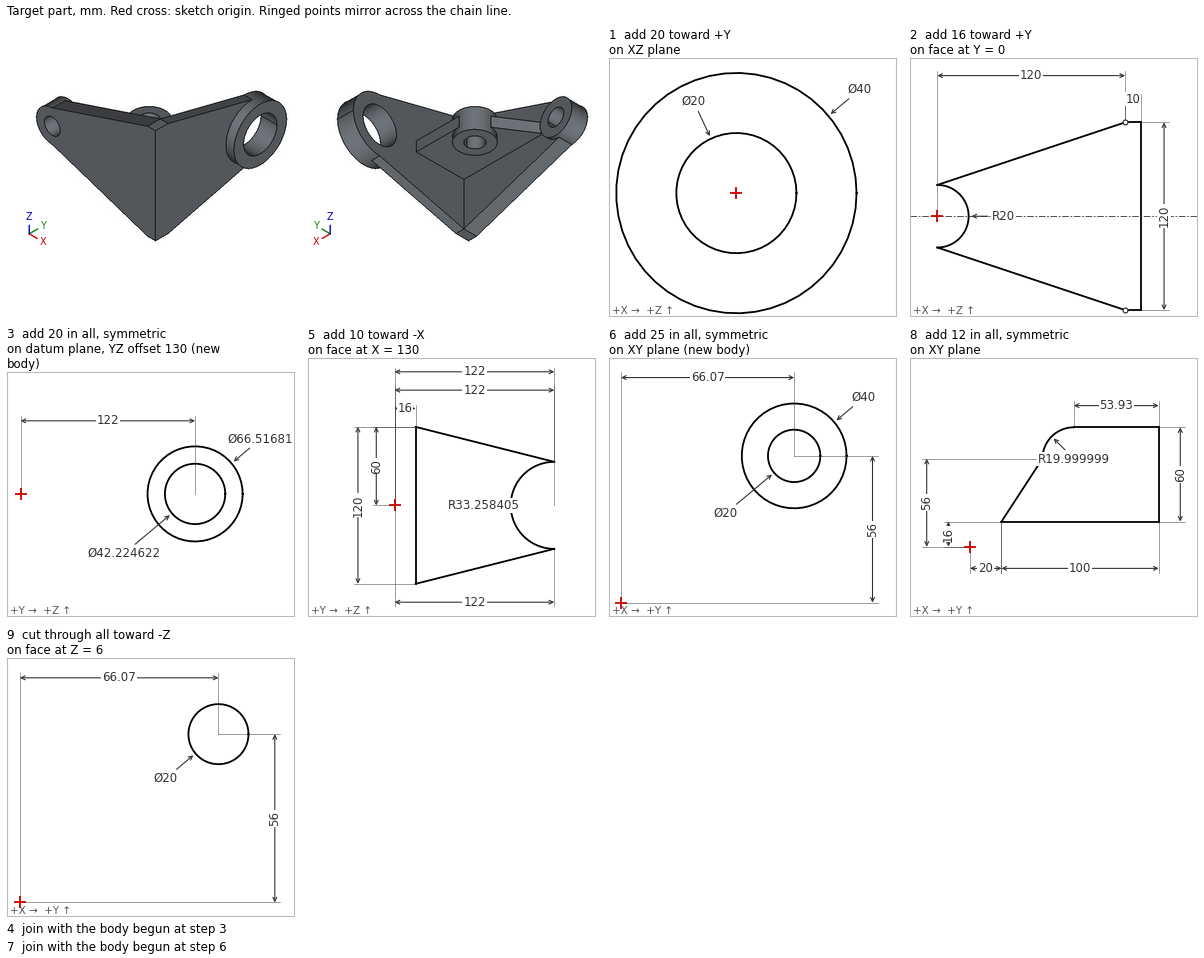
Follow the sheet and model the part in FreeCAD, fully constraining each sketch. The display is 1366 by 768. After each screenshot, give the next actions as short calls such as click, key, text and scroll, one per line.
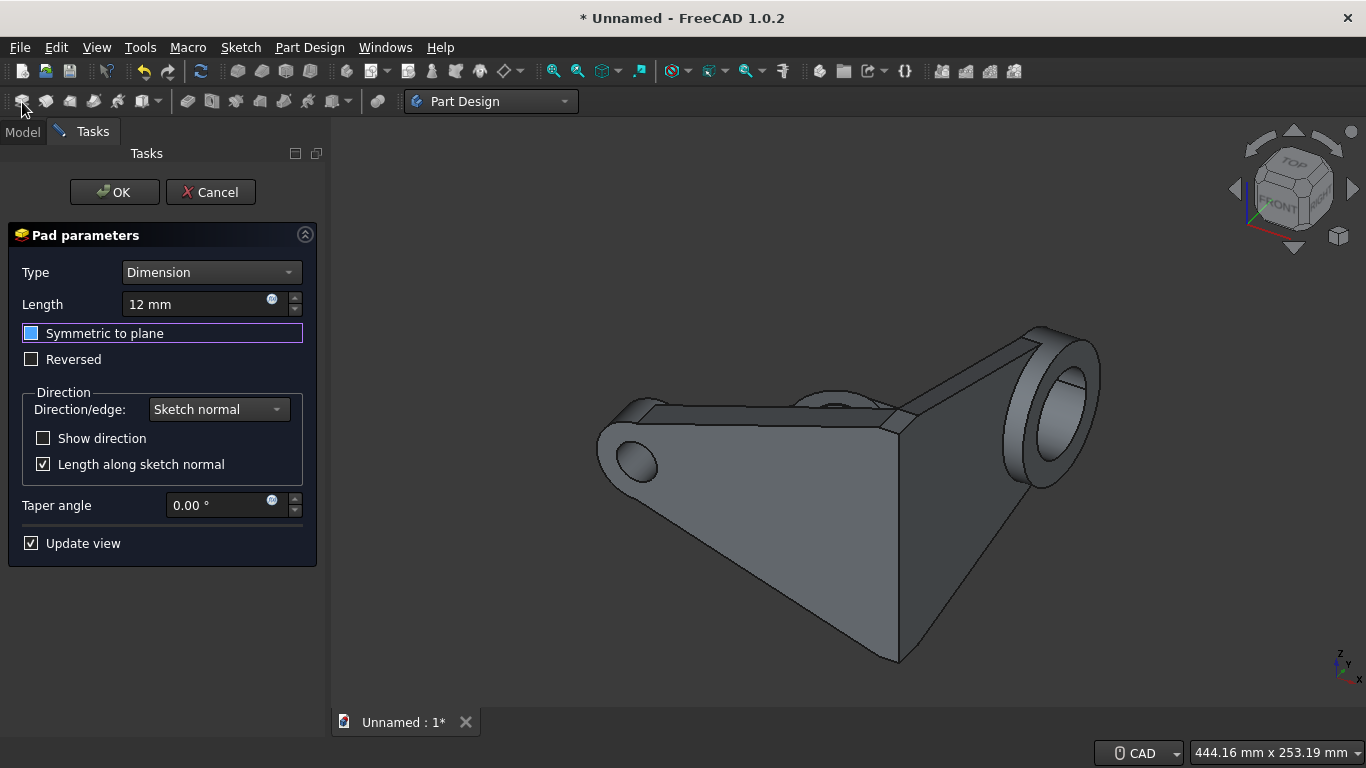
click(30, 333)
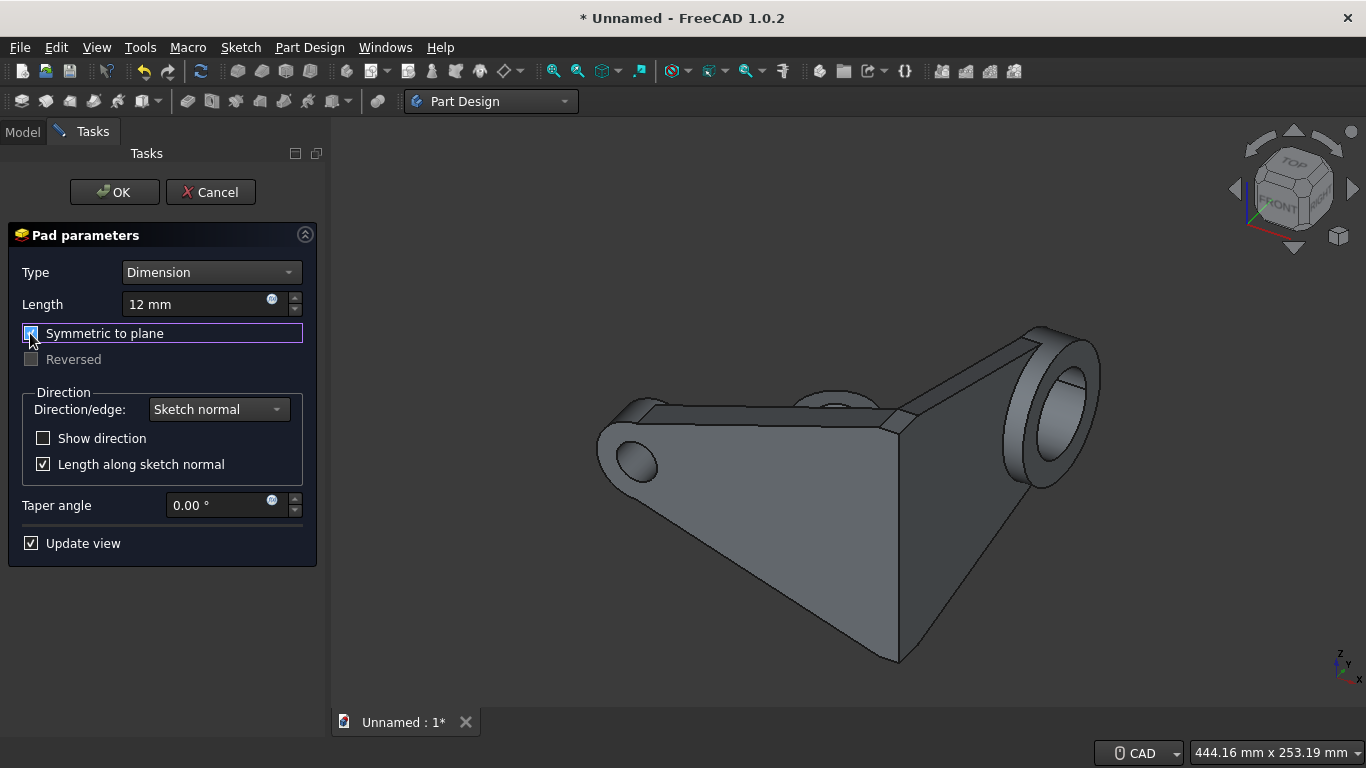
click(115, 192)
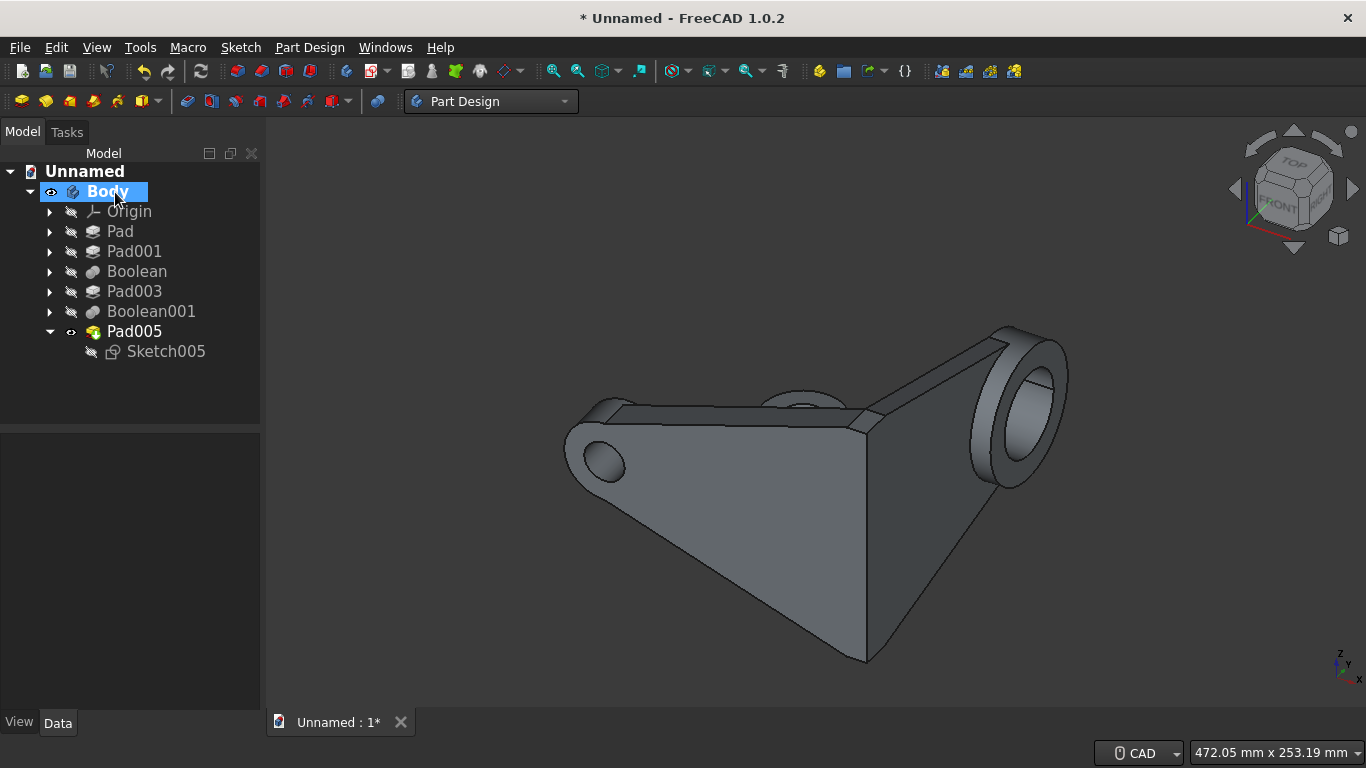
key(0)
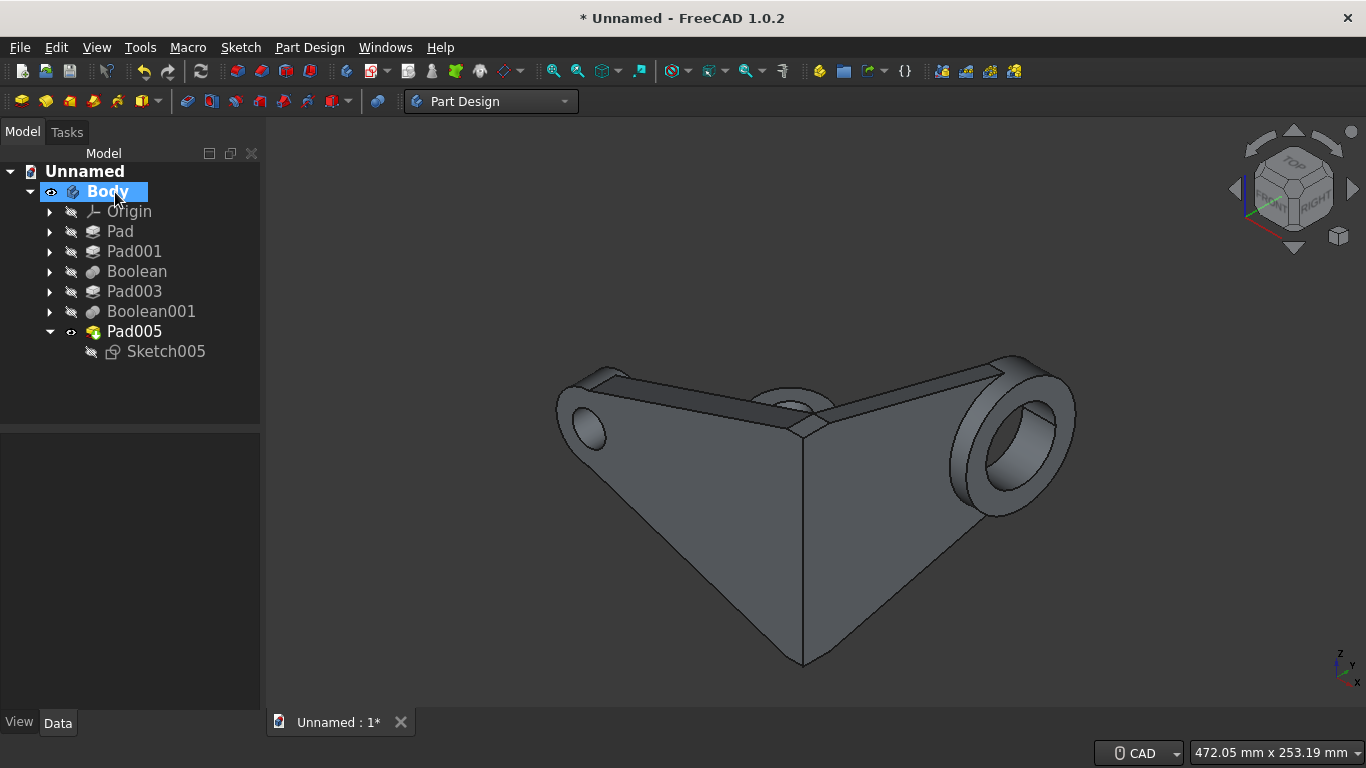
key(2)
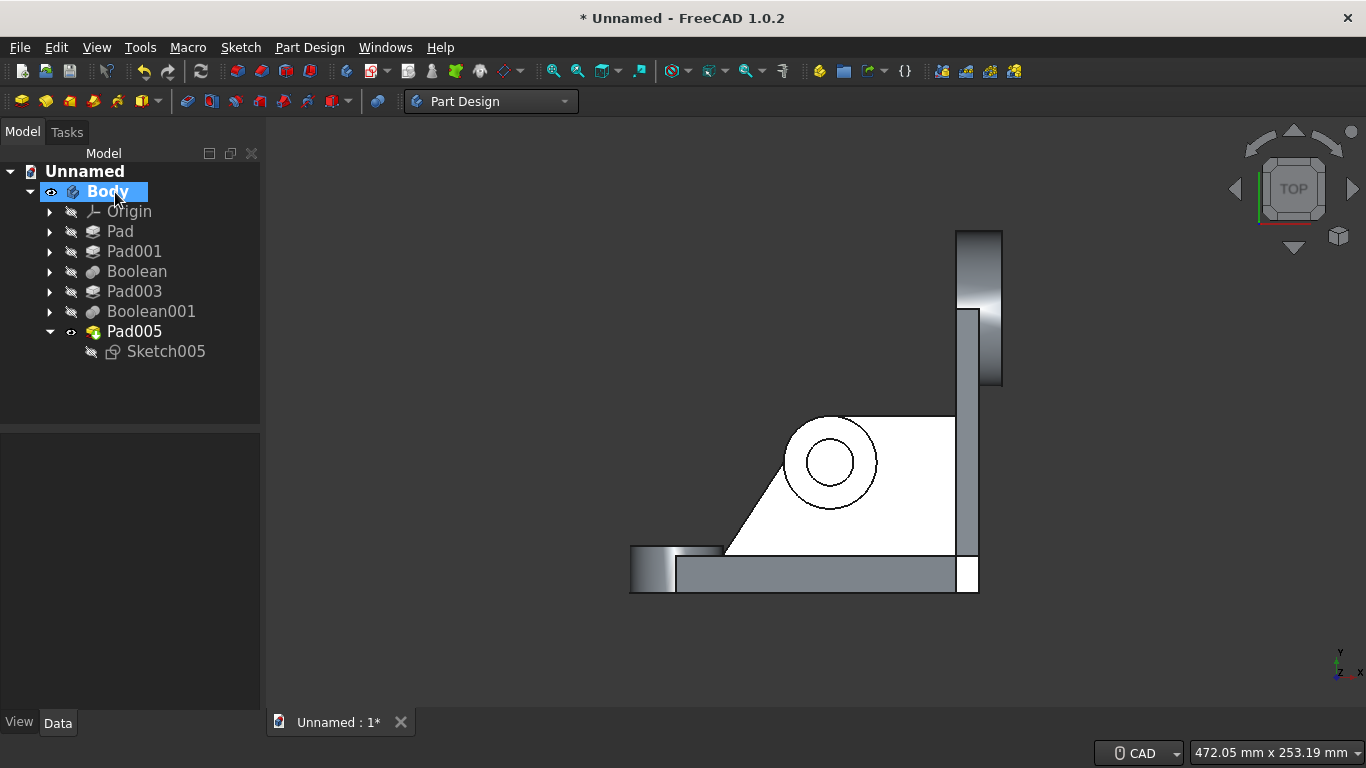
click(906, 505)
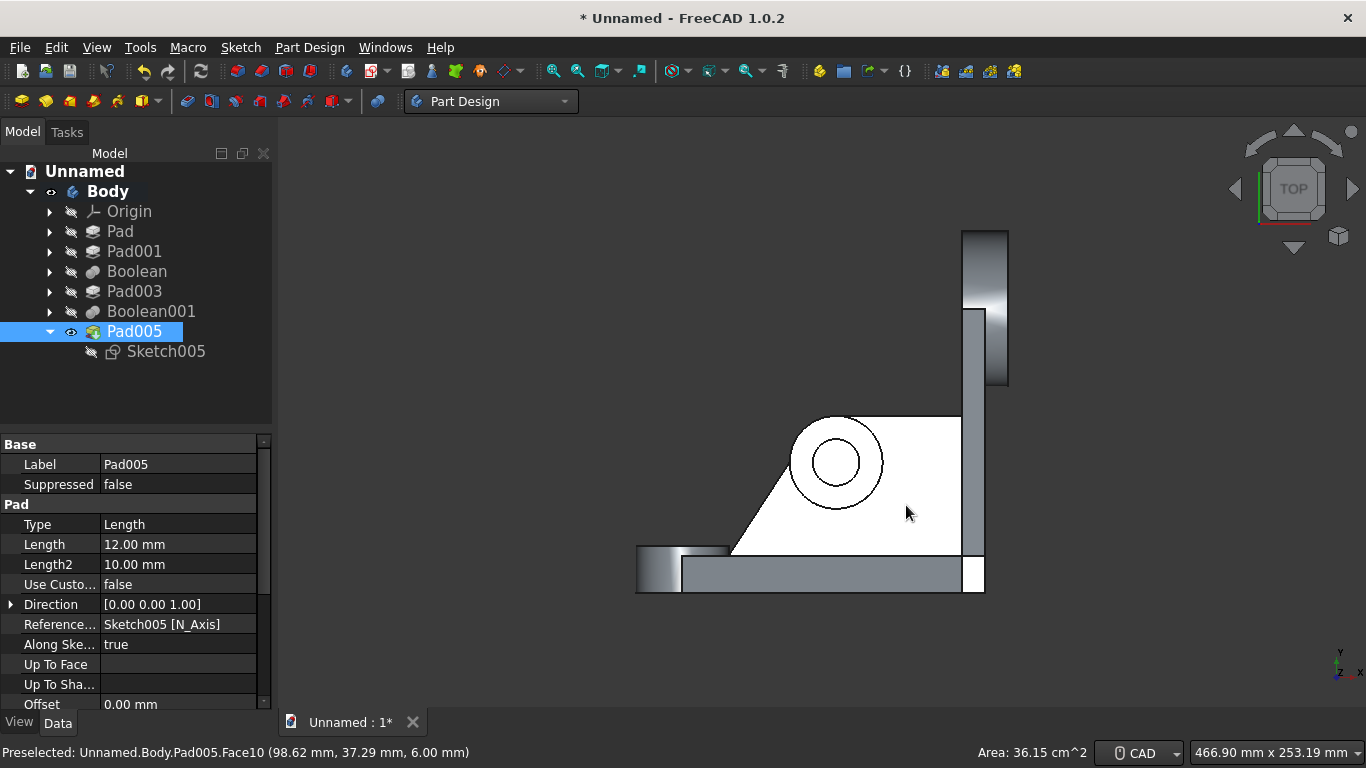
click(372, 72)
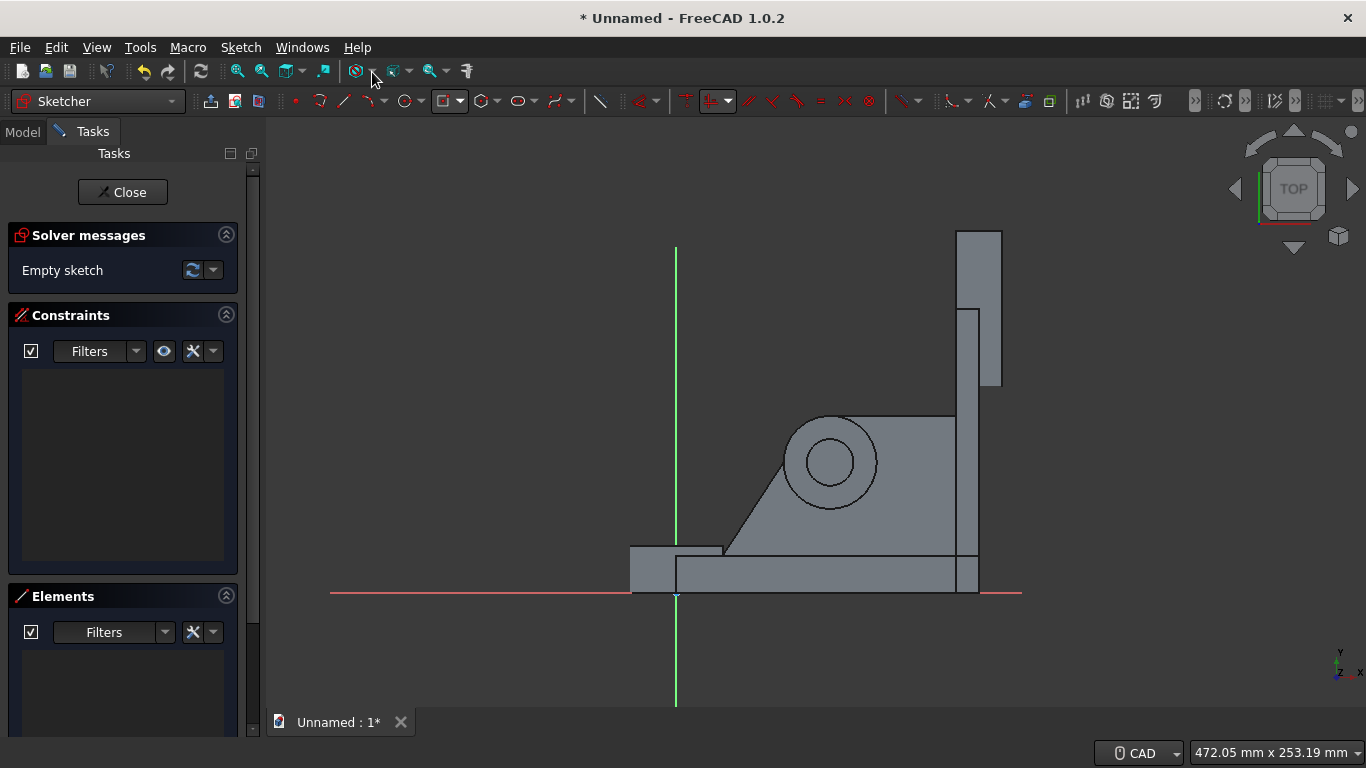
scroll(843, 470, up, 10)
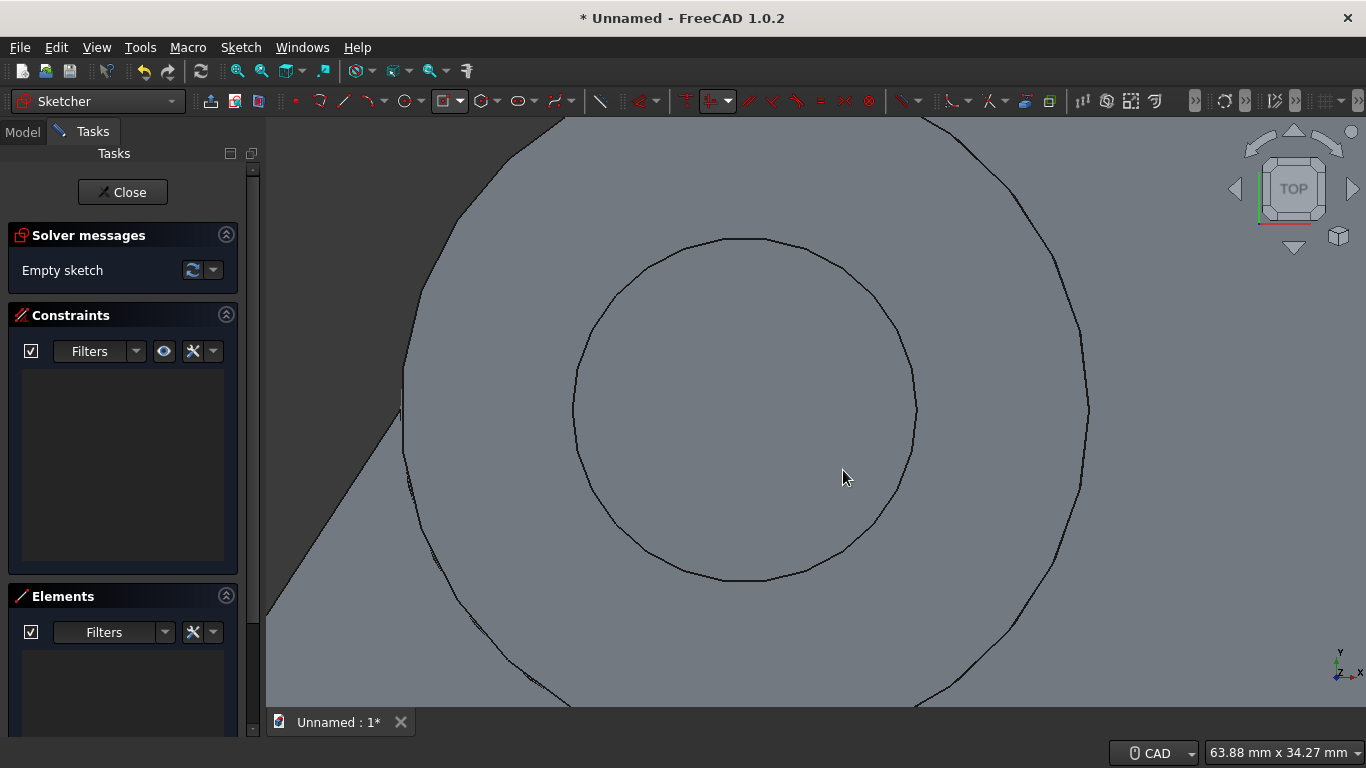
key(g)
key(c)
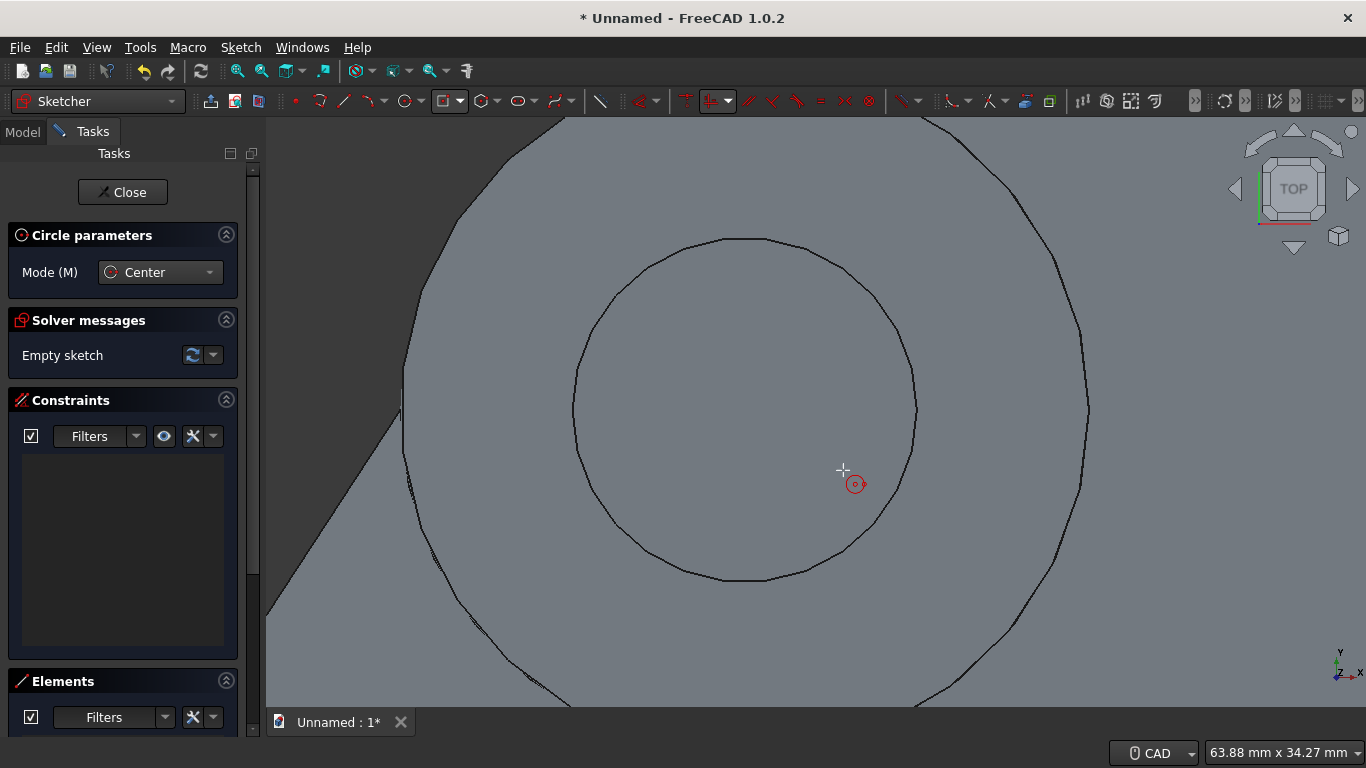
click(745, 410)
click(866, 288)
key(Escape)